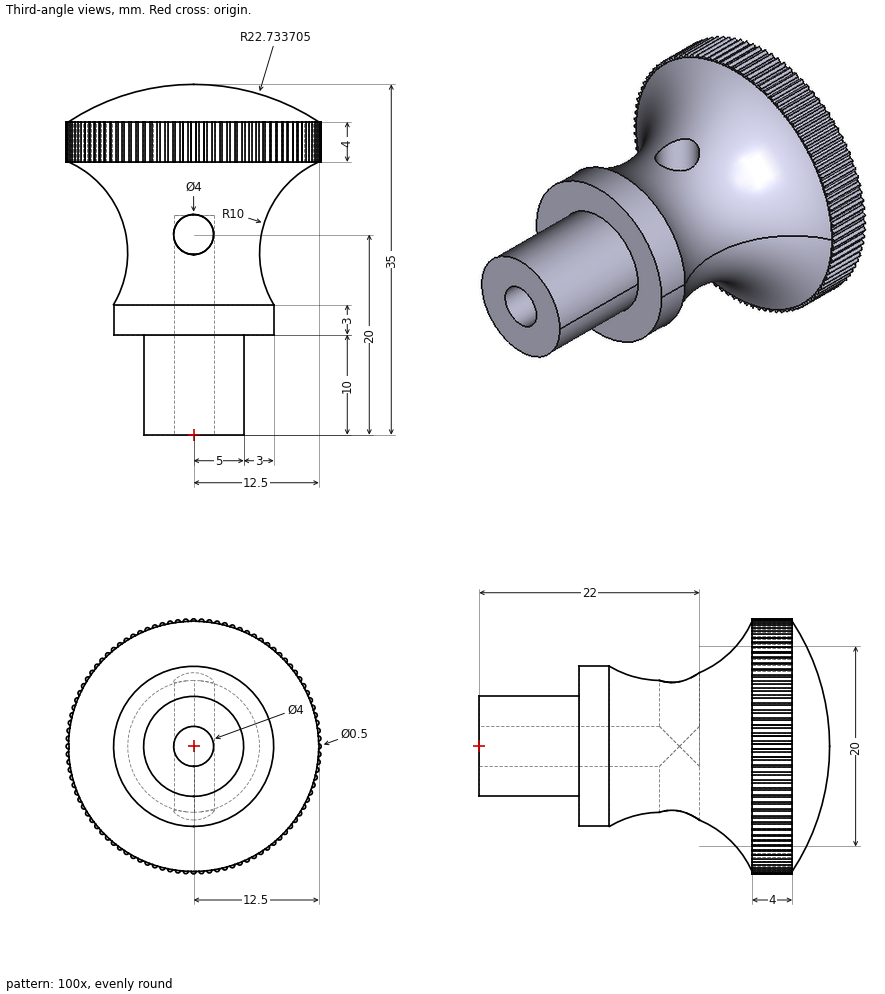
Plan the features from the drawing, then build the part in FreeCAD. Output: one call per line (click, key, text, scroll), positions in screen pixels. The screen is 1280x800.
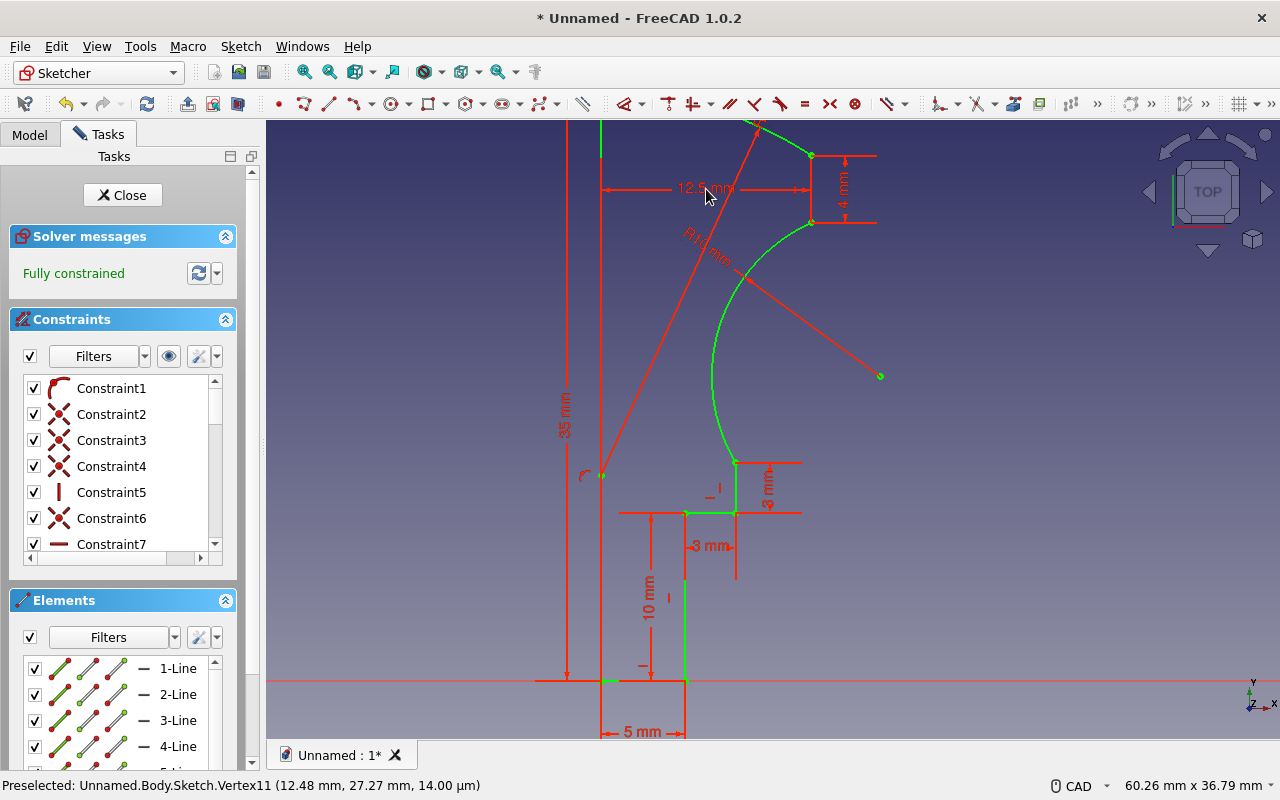
click(123, 195)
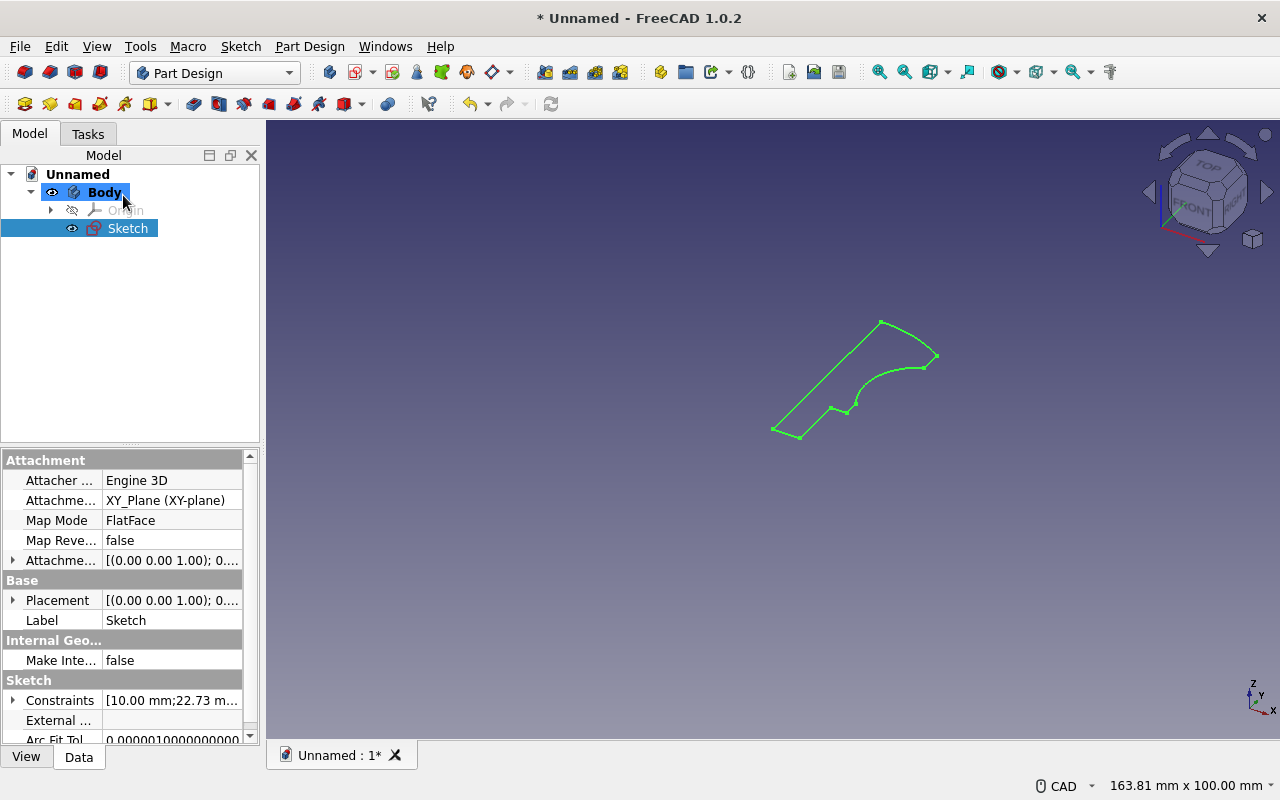
click(50, 104)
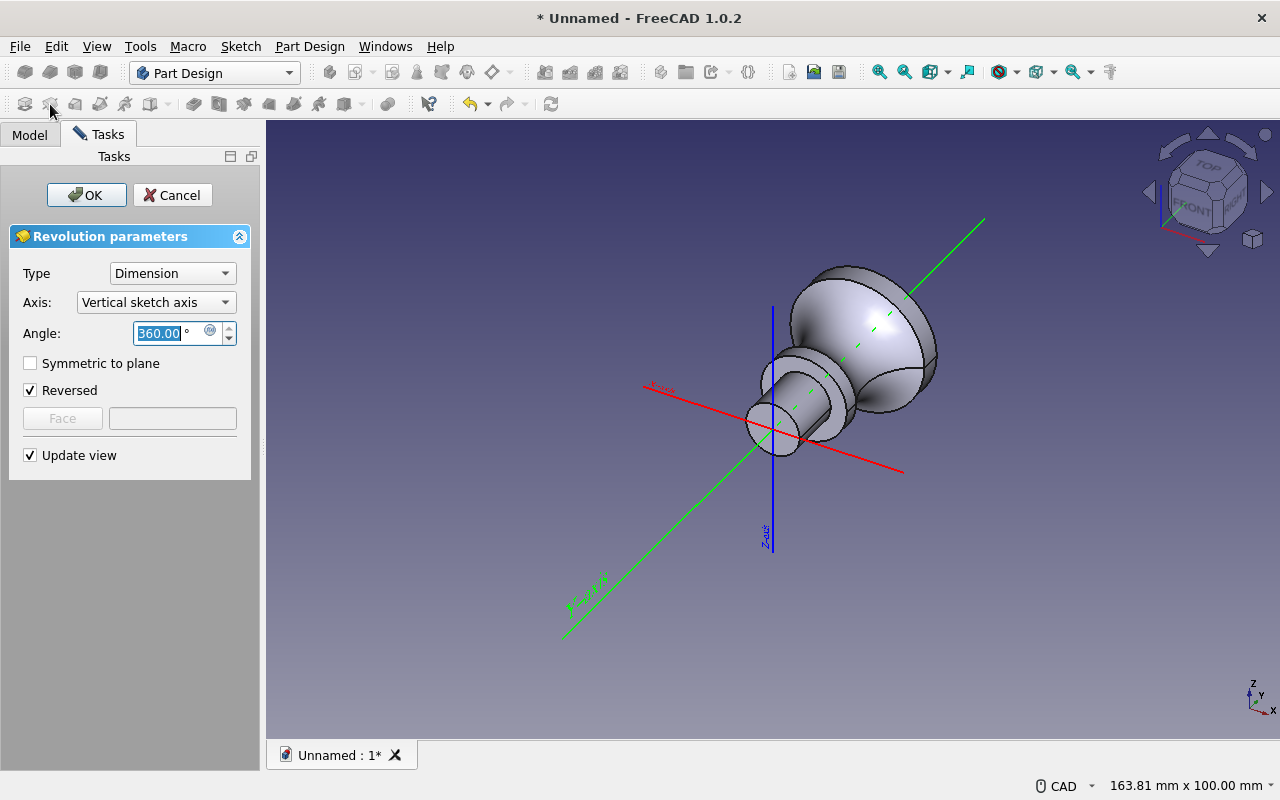
click(87, 195)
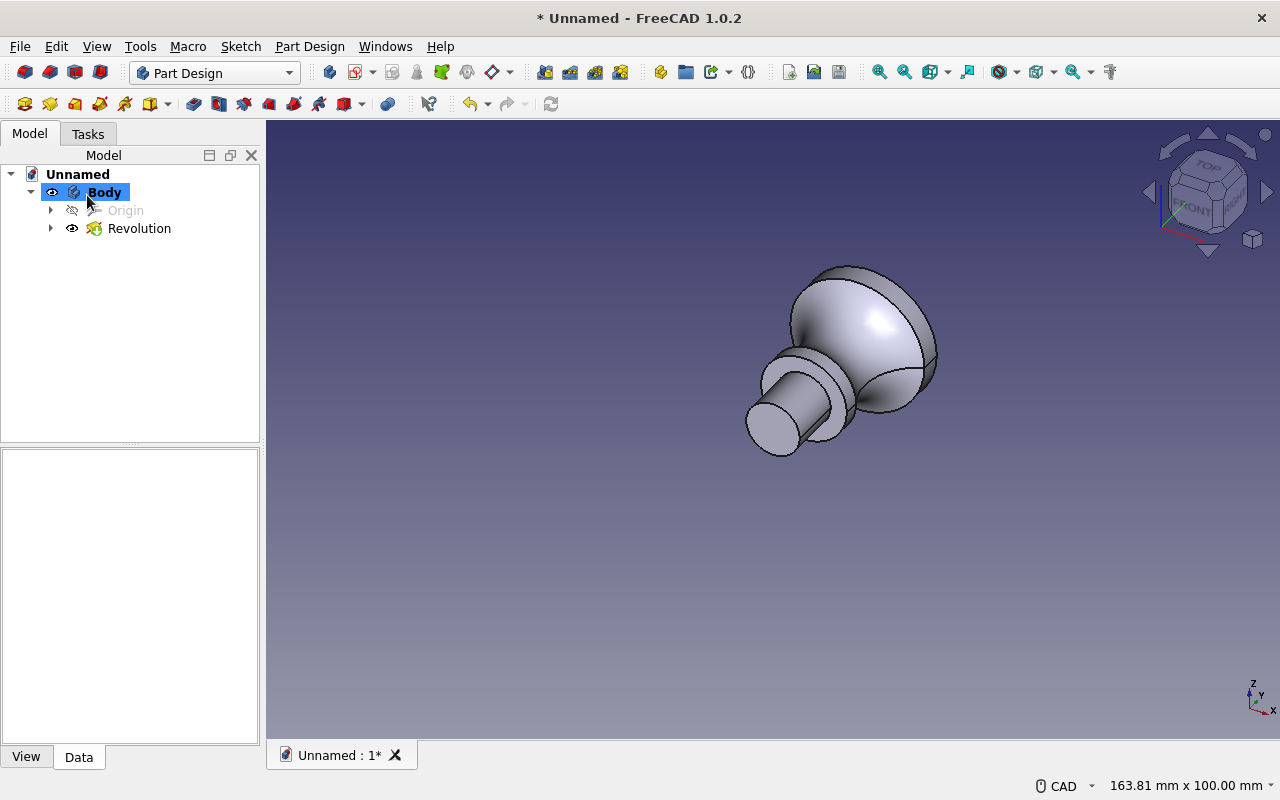
click(354, 72)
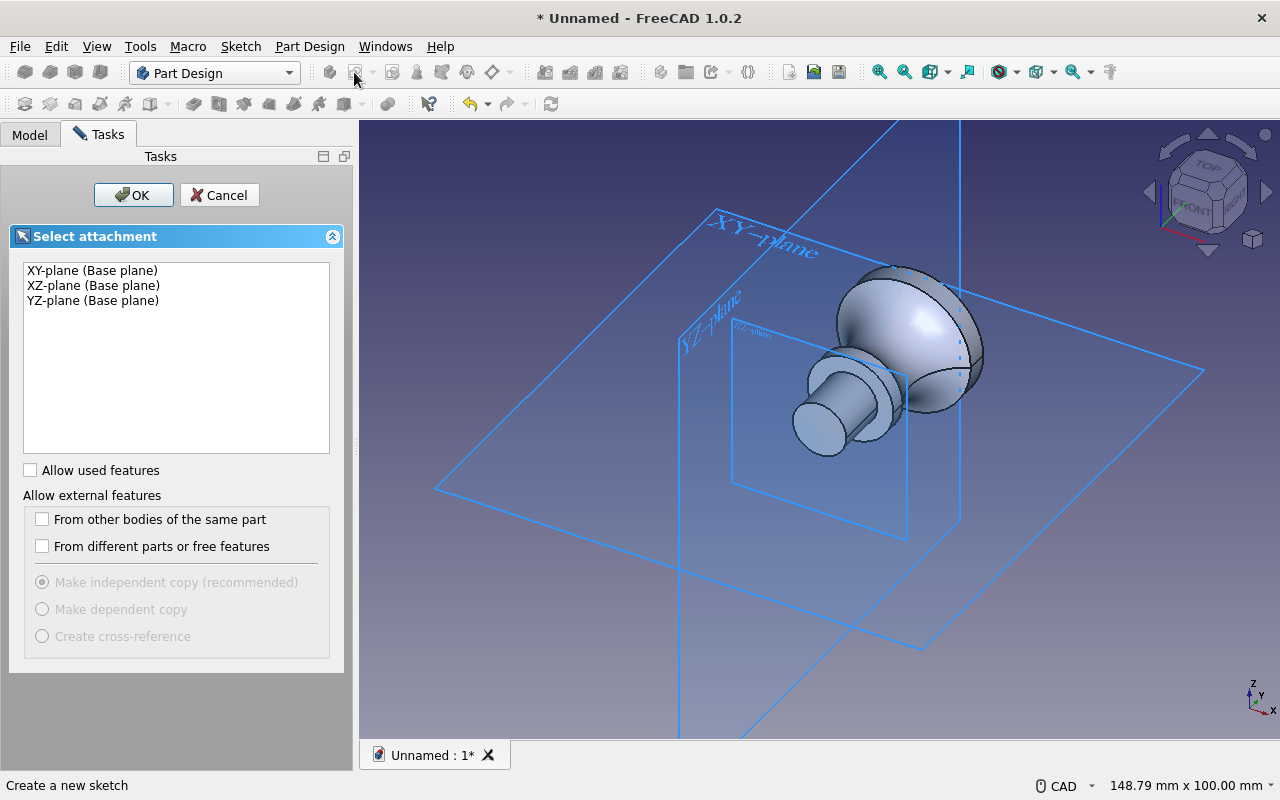
click(84, 270)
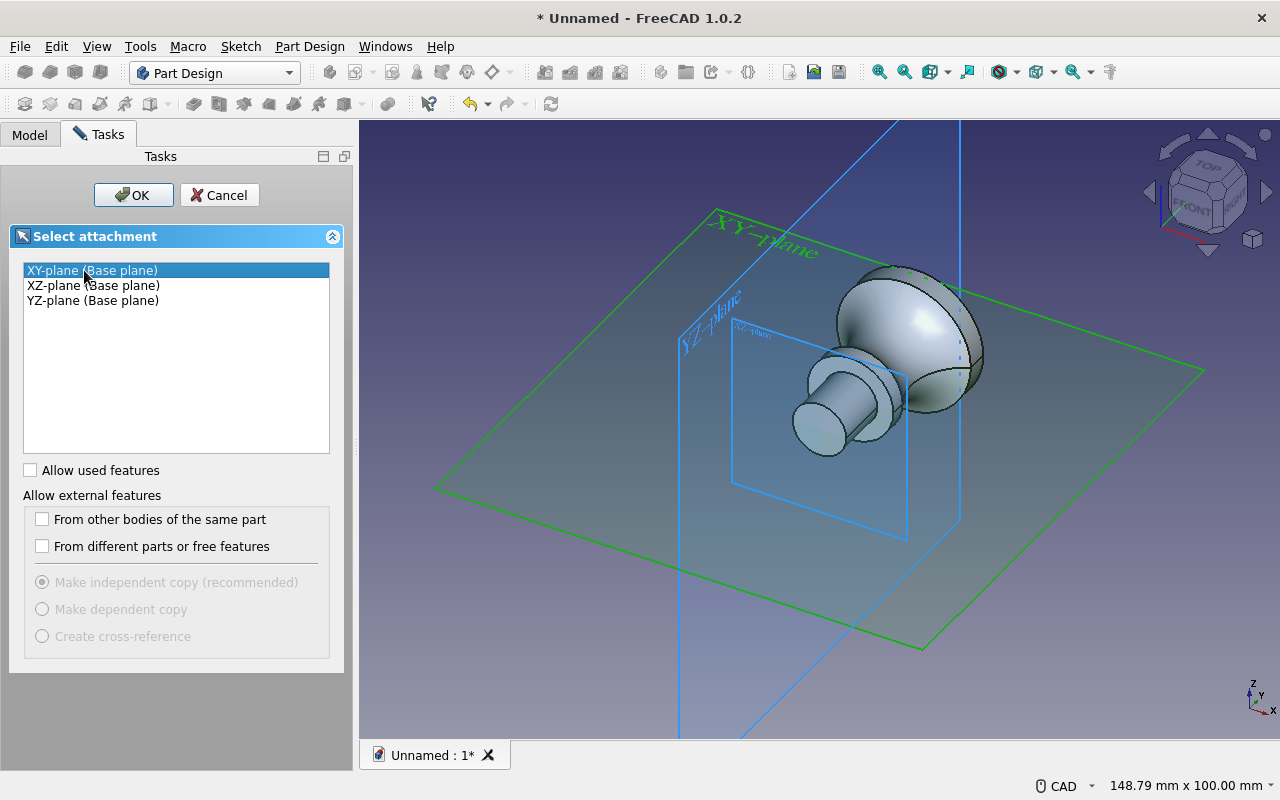
click(134, 195)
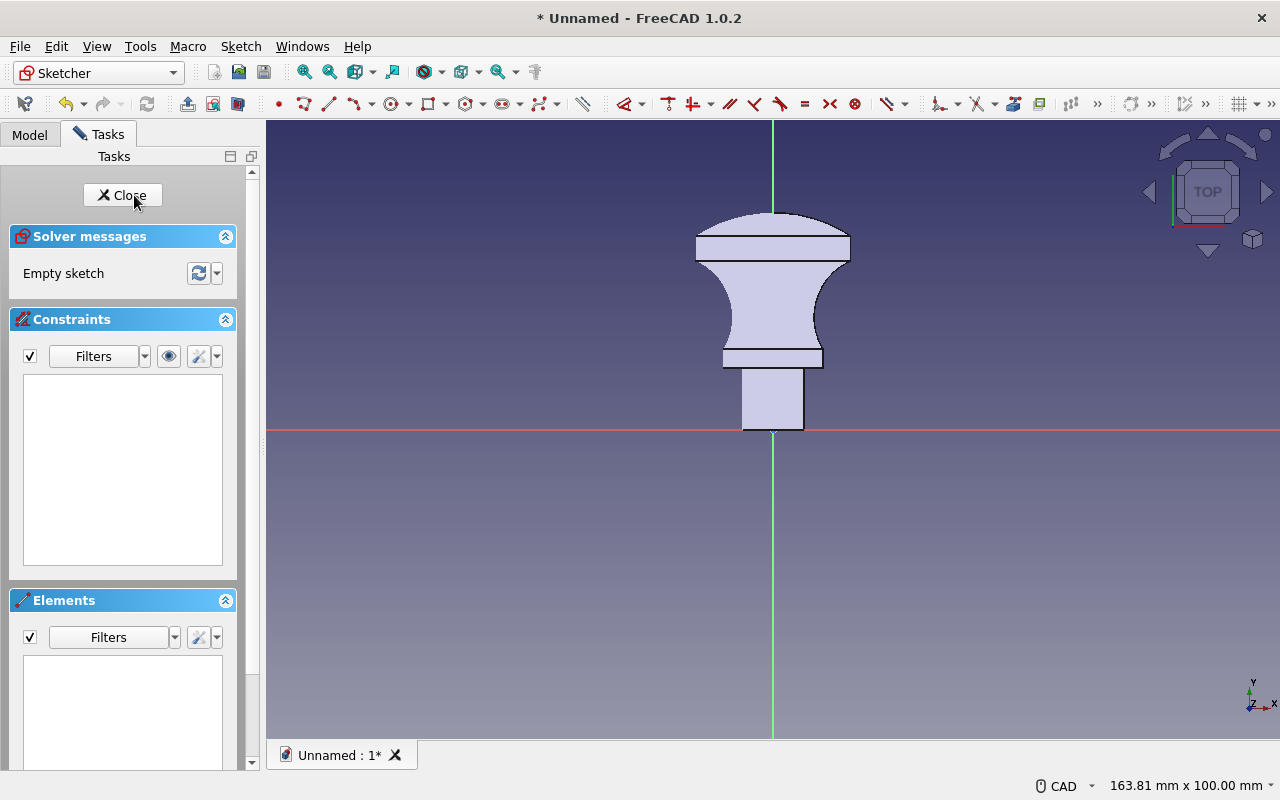
click(238, 104)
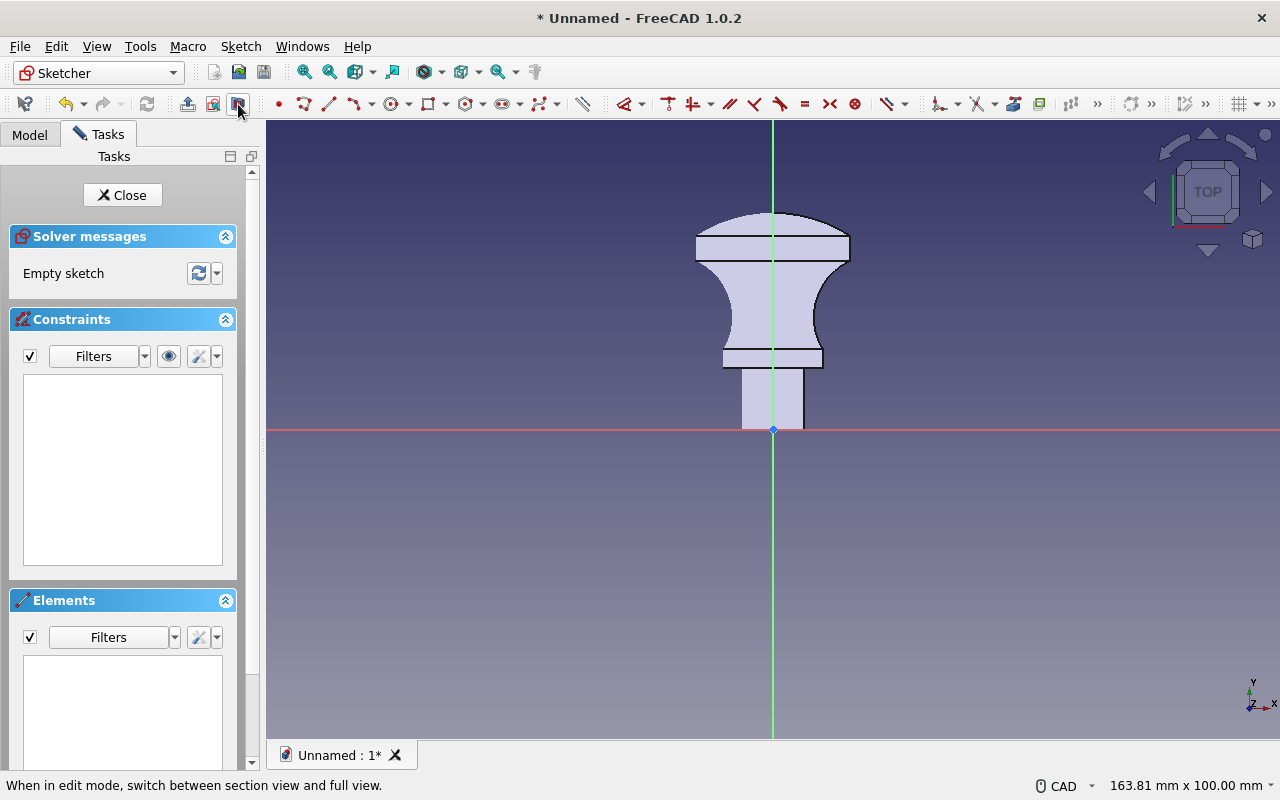
scroll(777, 298, up, 14)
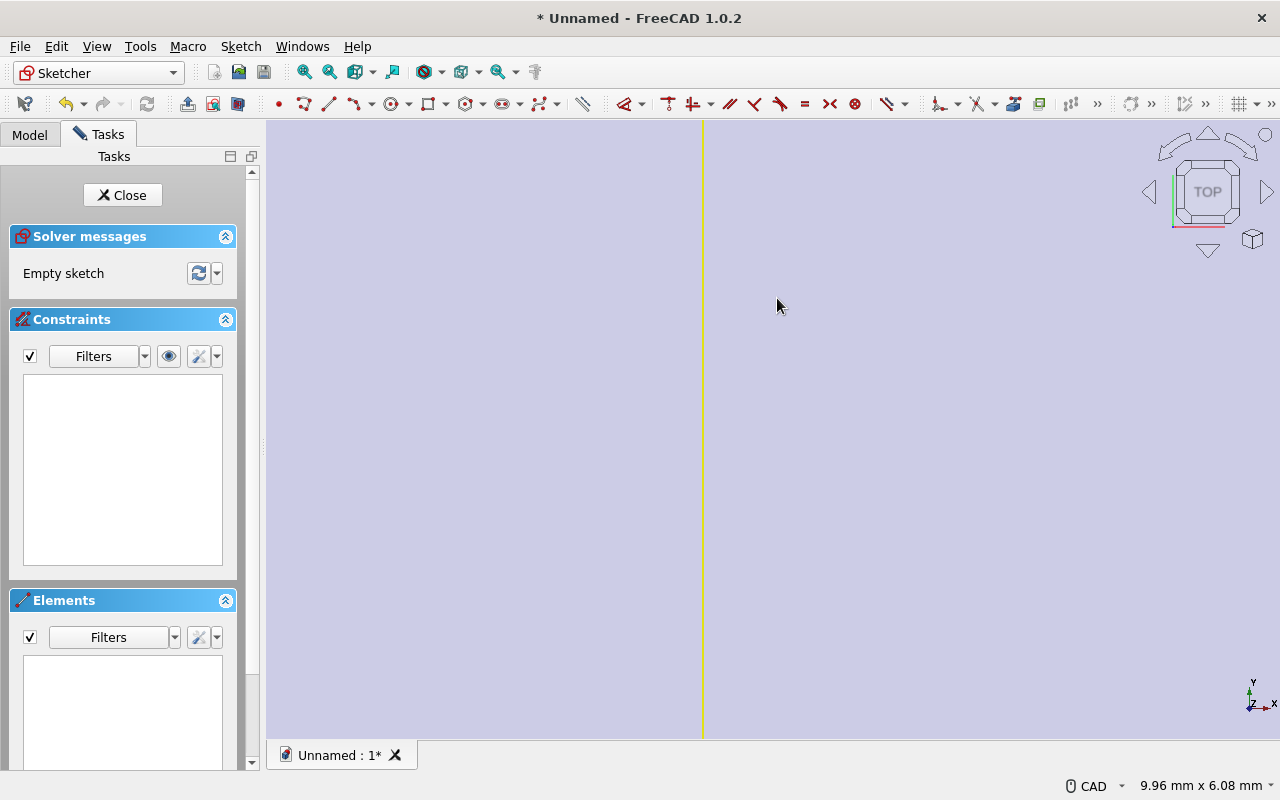
click(390, 104)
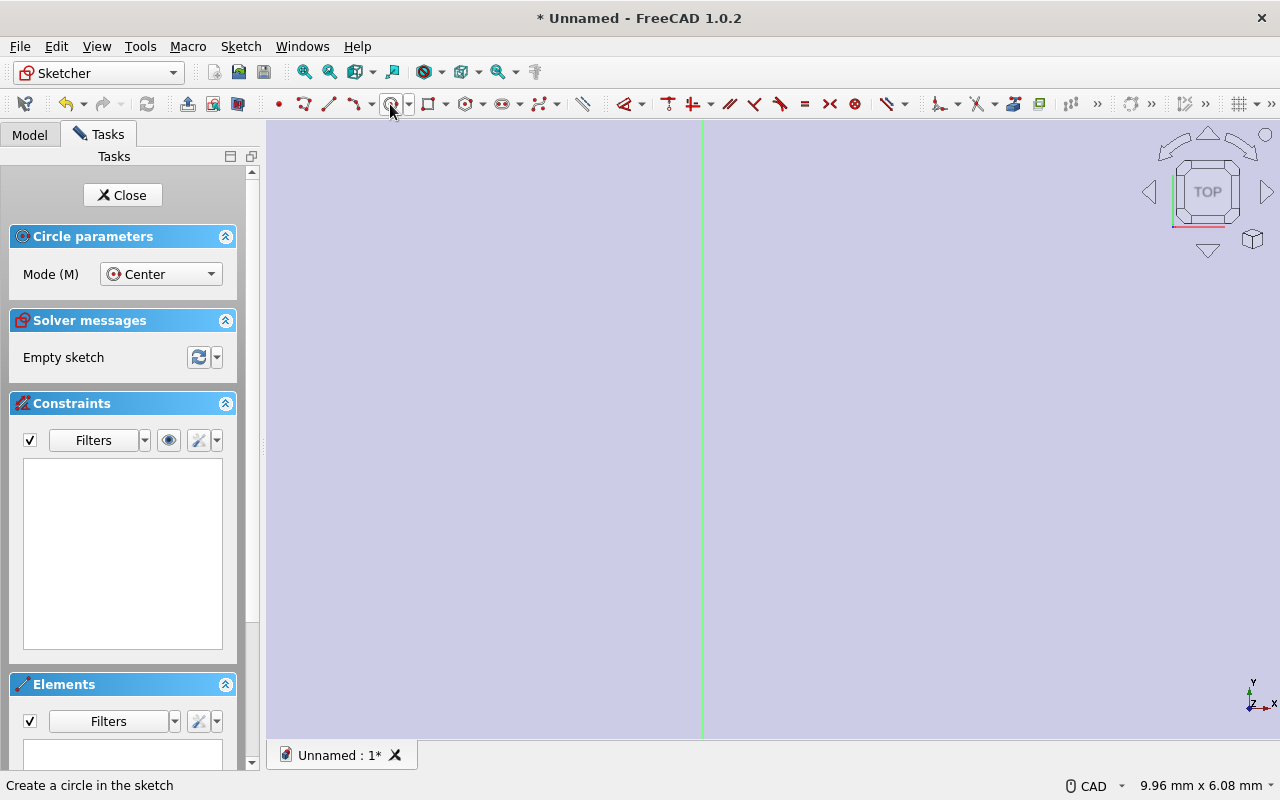
click(703, 420)
move(847, 276)